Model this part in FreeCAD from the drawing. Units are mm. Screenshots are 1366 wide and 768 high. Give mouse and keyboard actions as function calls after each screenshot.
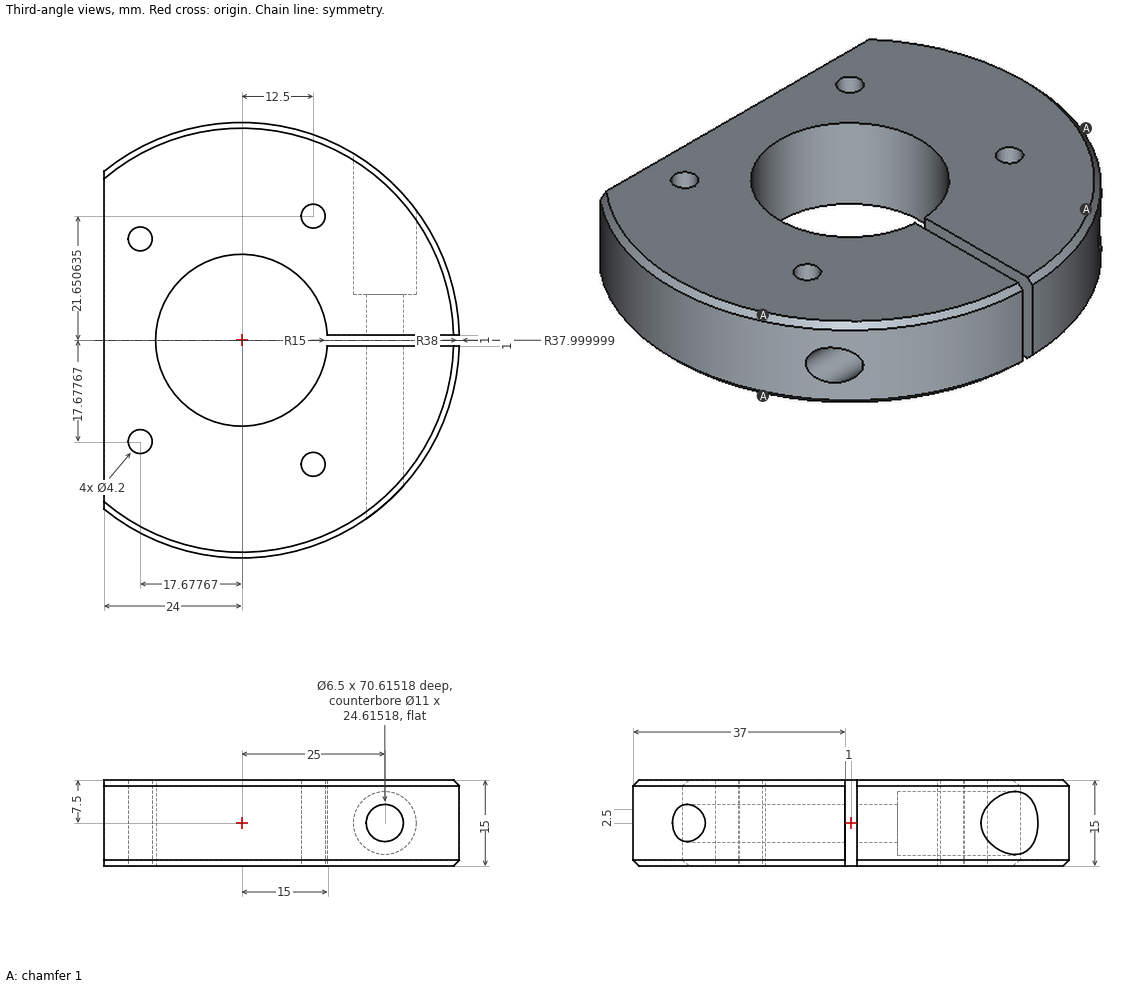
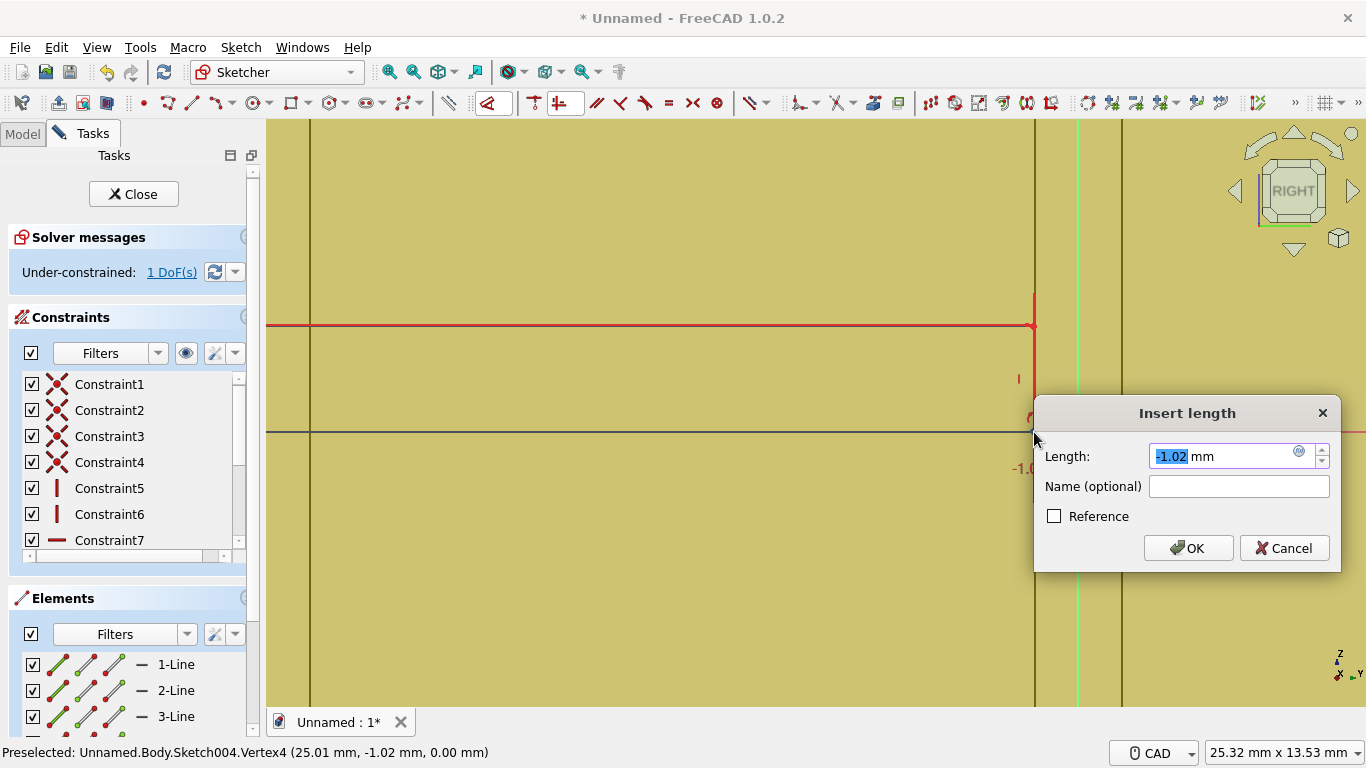
text(-1)
key(Return)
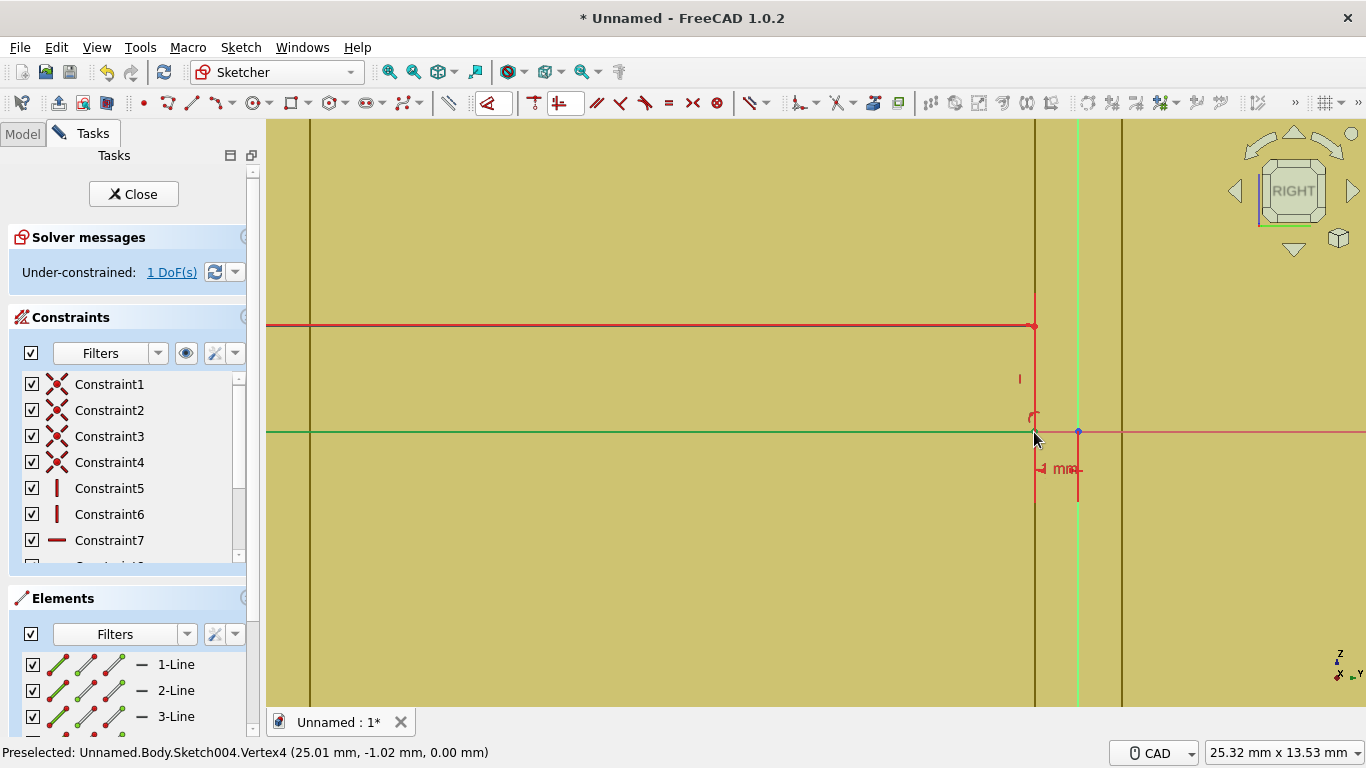
scroll(1035, 434, down, 5)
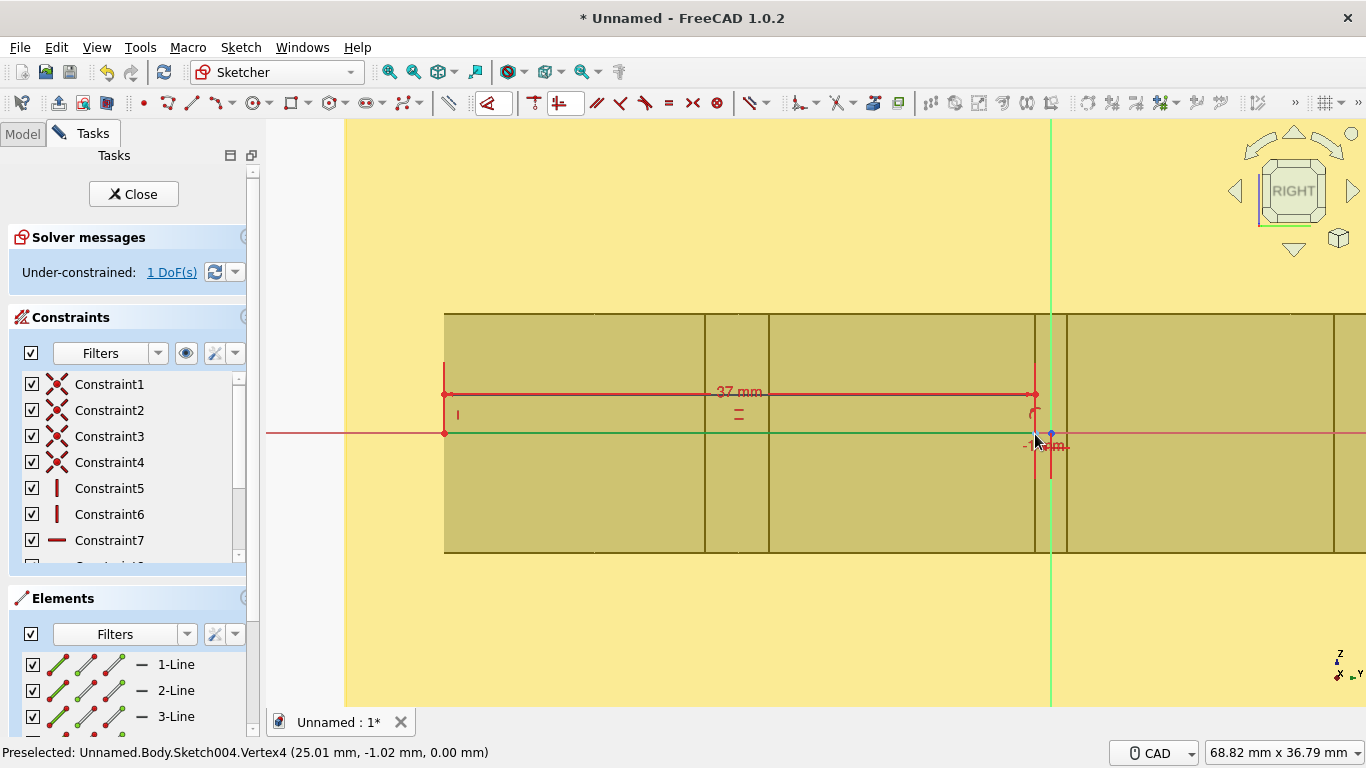
click(444, 406)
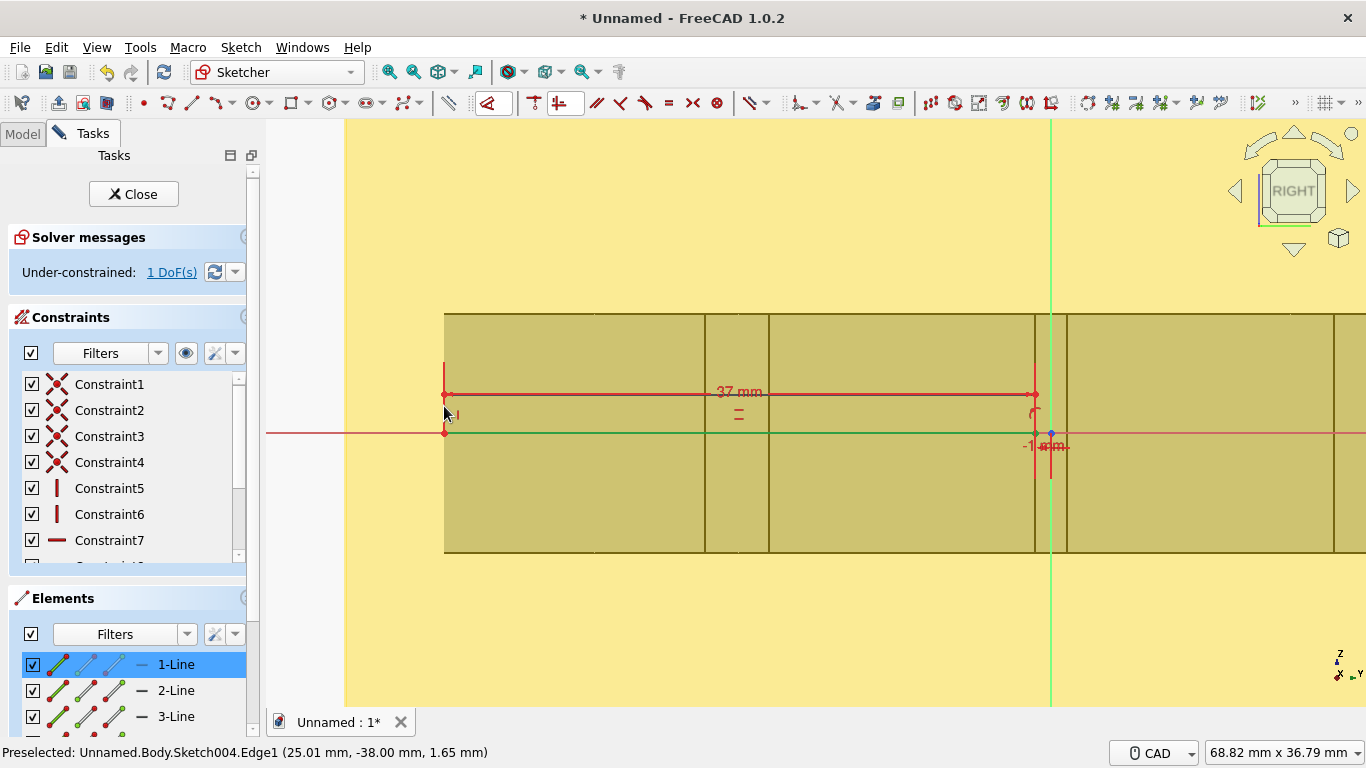
key(i)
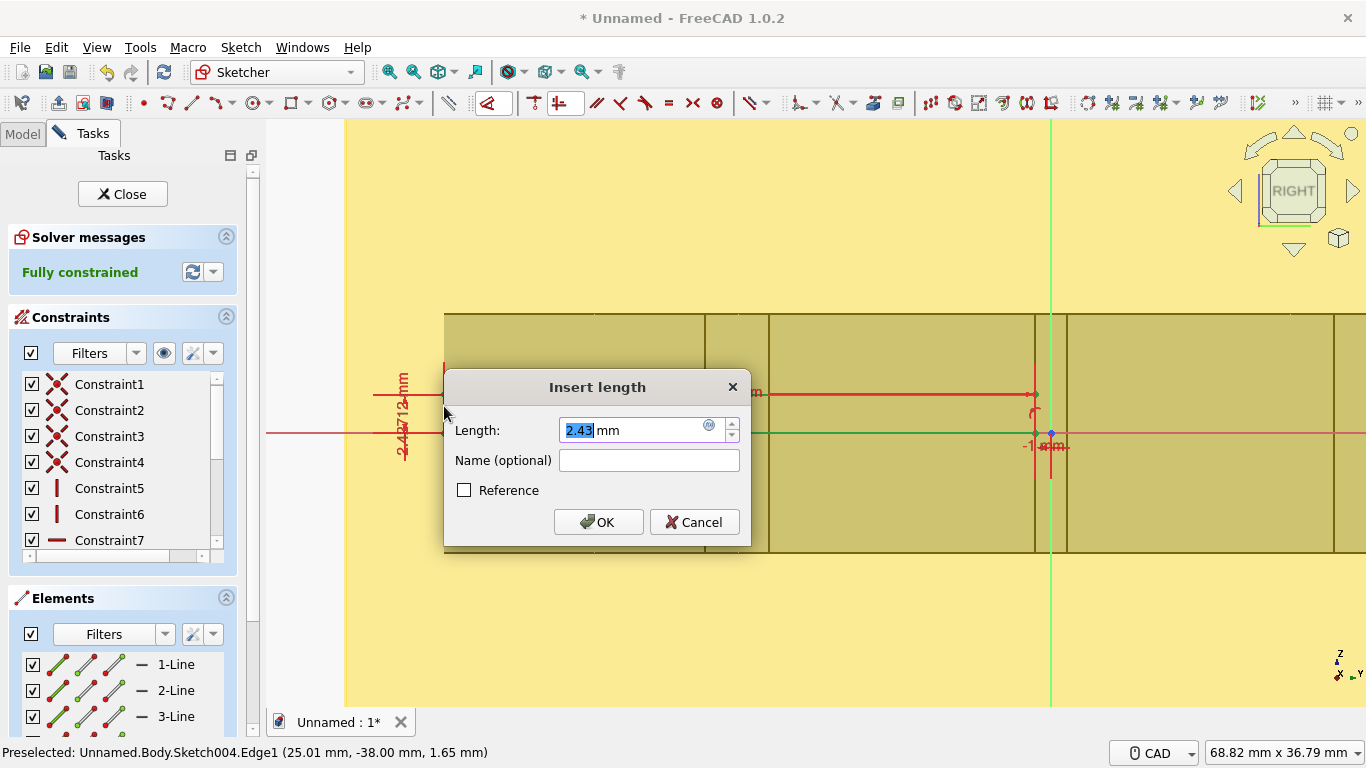
text(2.5)
key(Return)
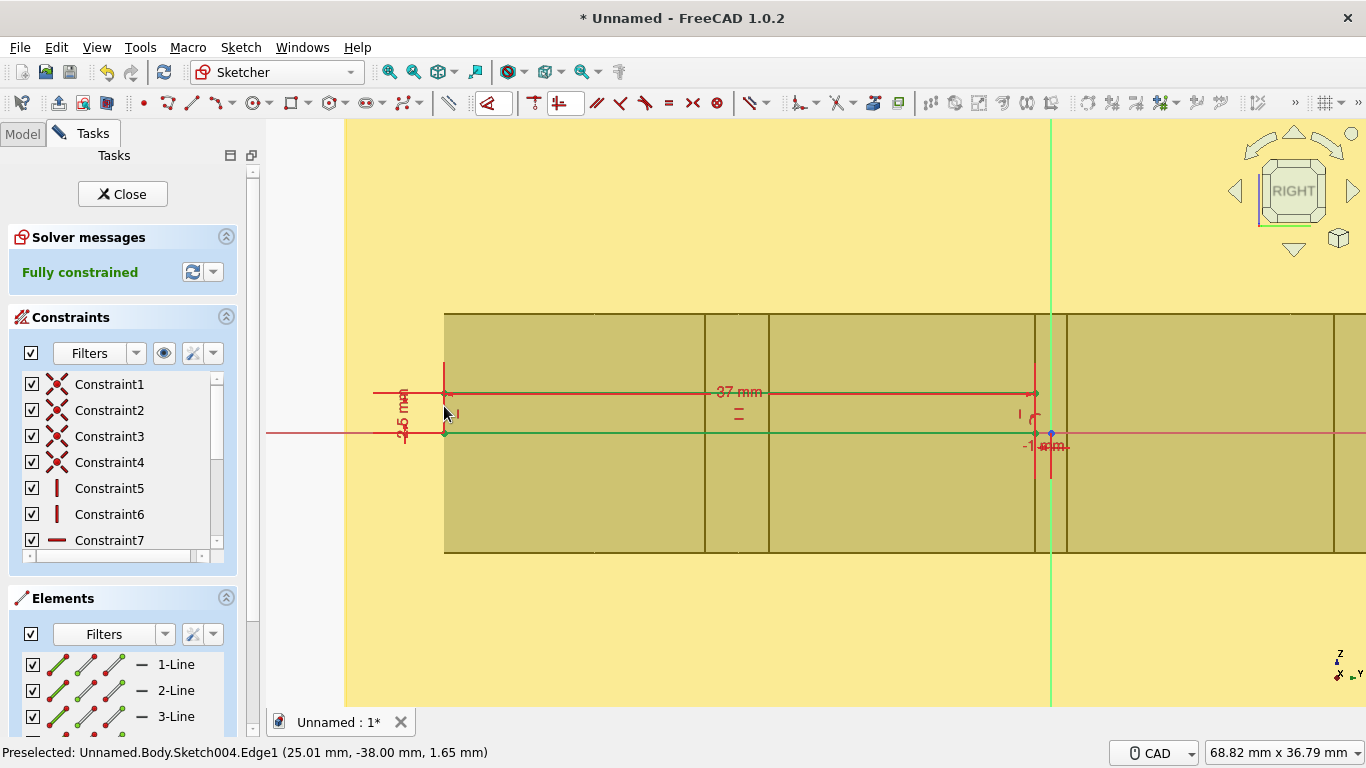
click(123, 194)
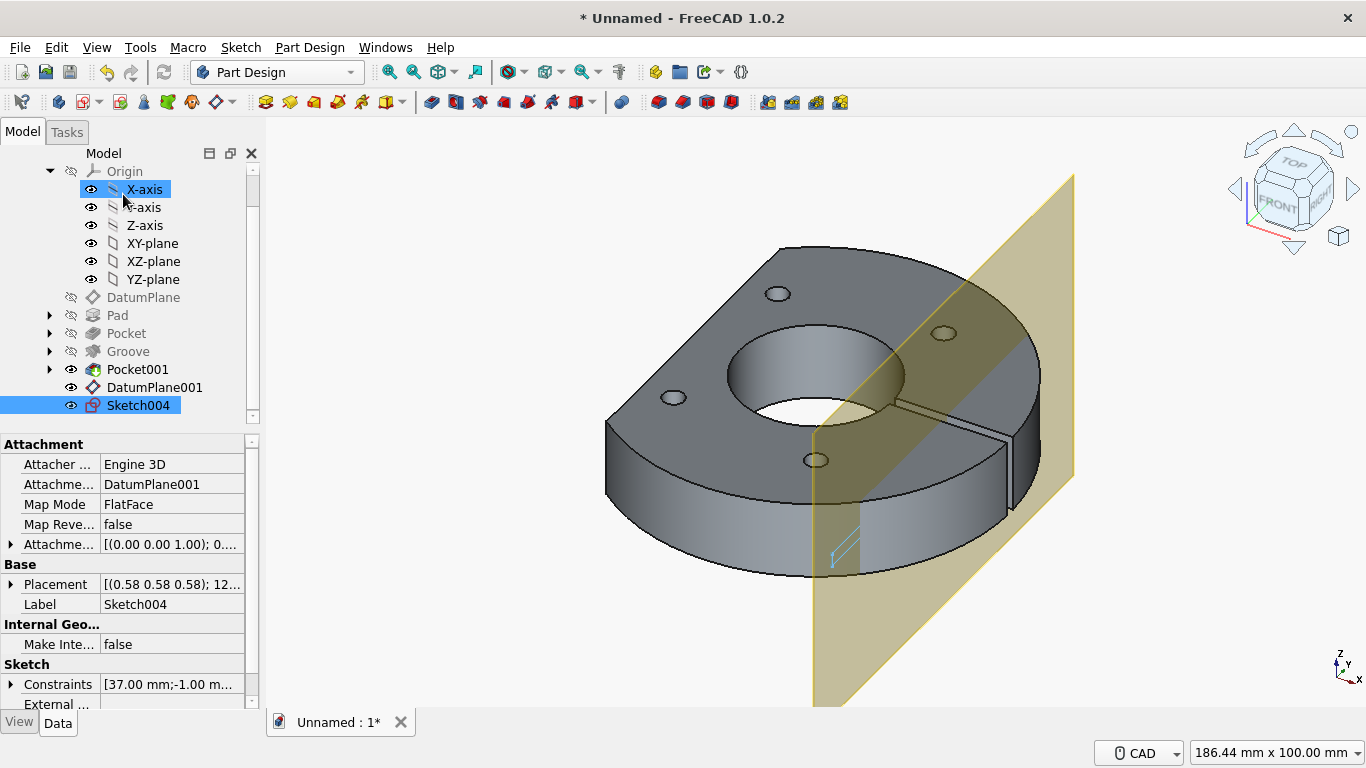
click(480, 102)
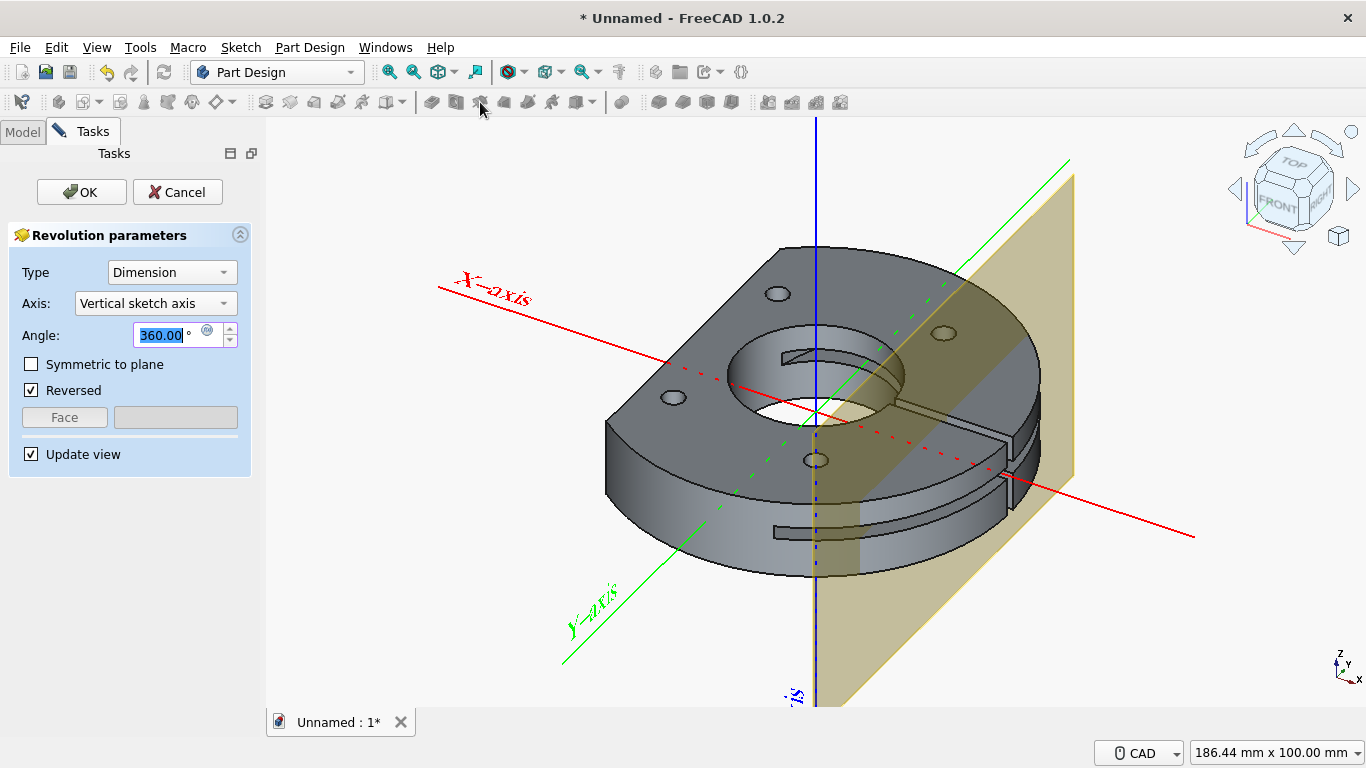
click(156, 304)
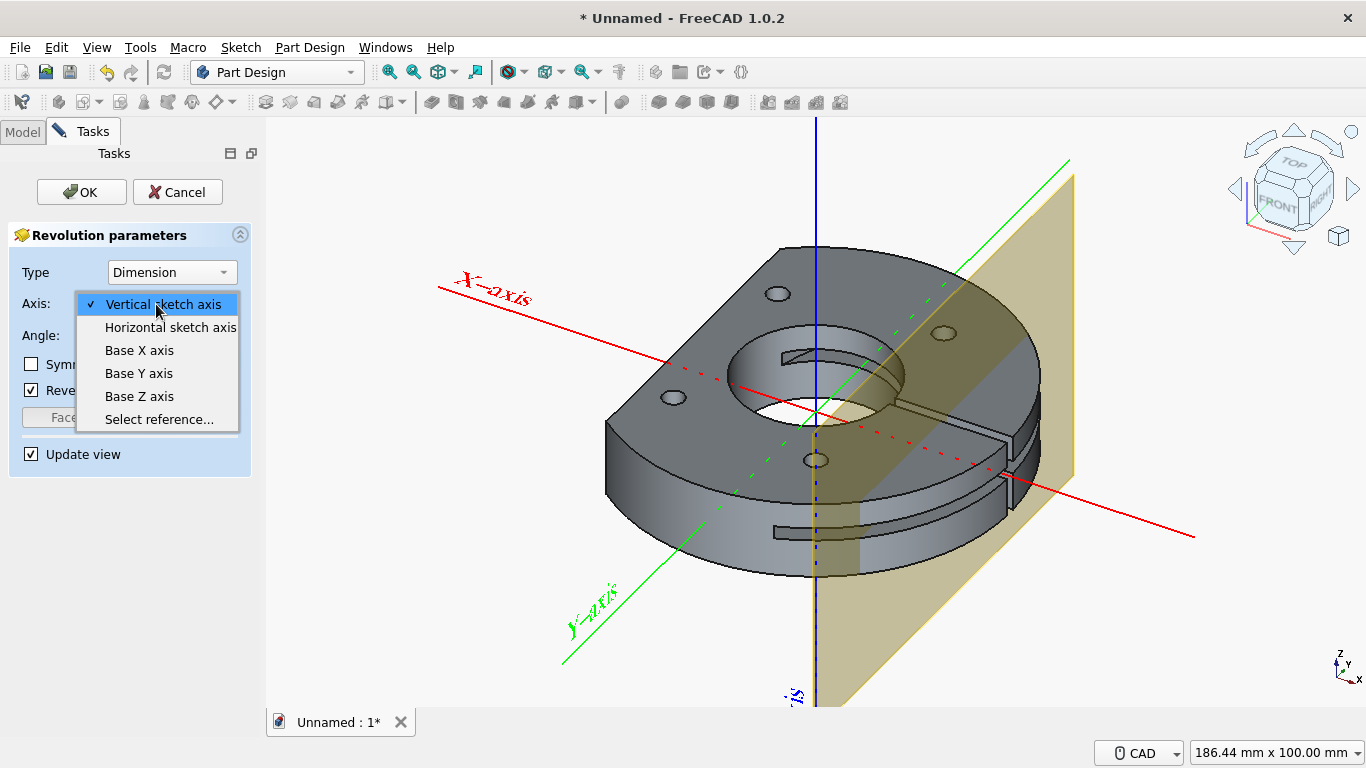
click(156, 328)